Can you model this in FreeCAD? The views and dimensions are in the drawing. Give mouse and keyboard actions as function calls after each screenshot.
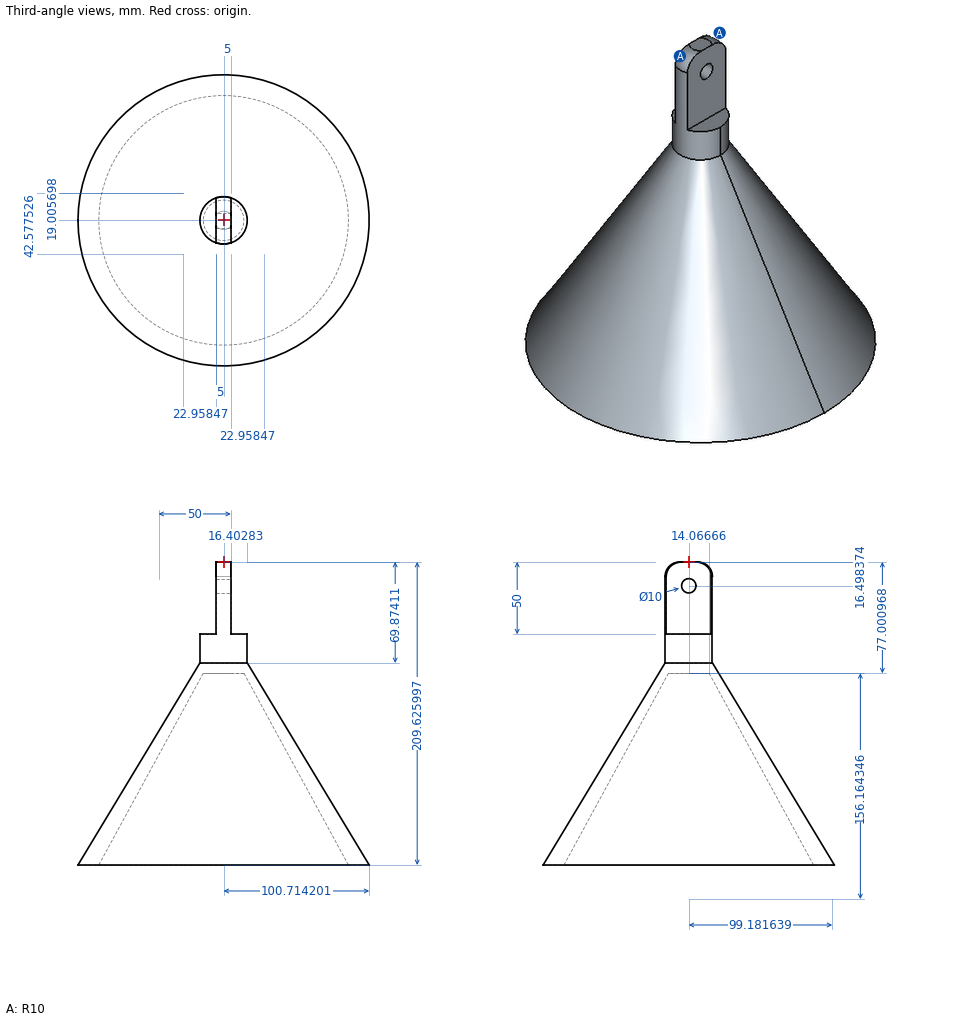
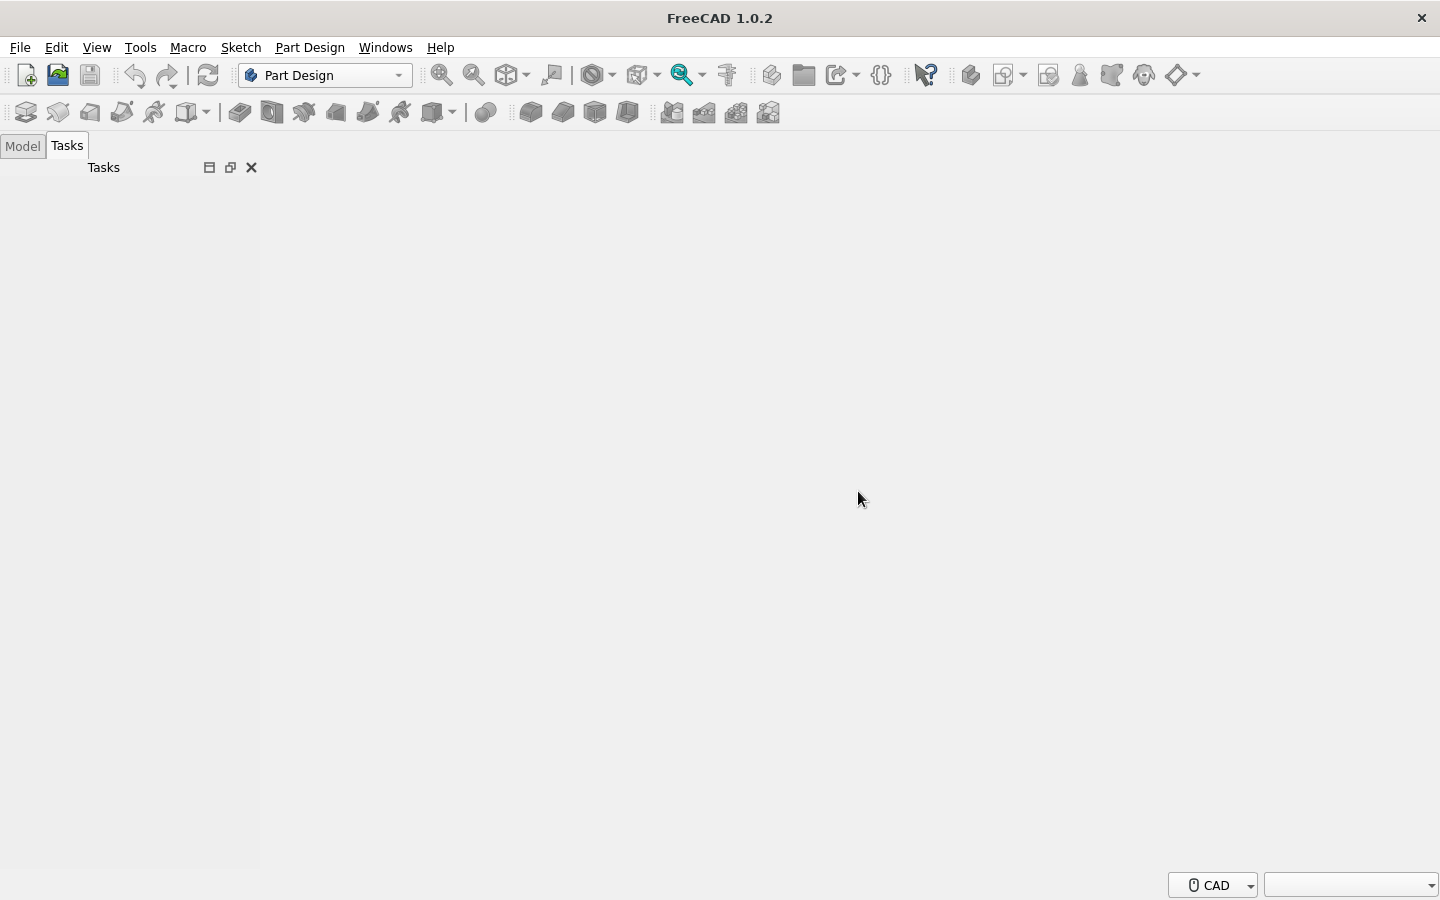
click(26, 76)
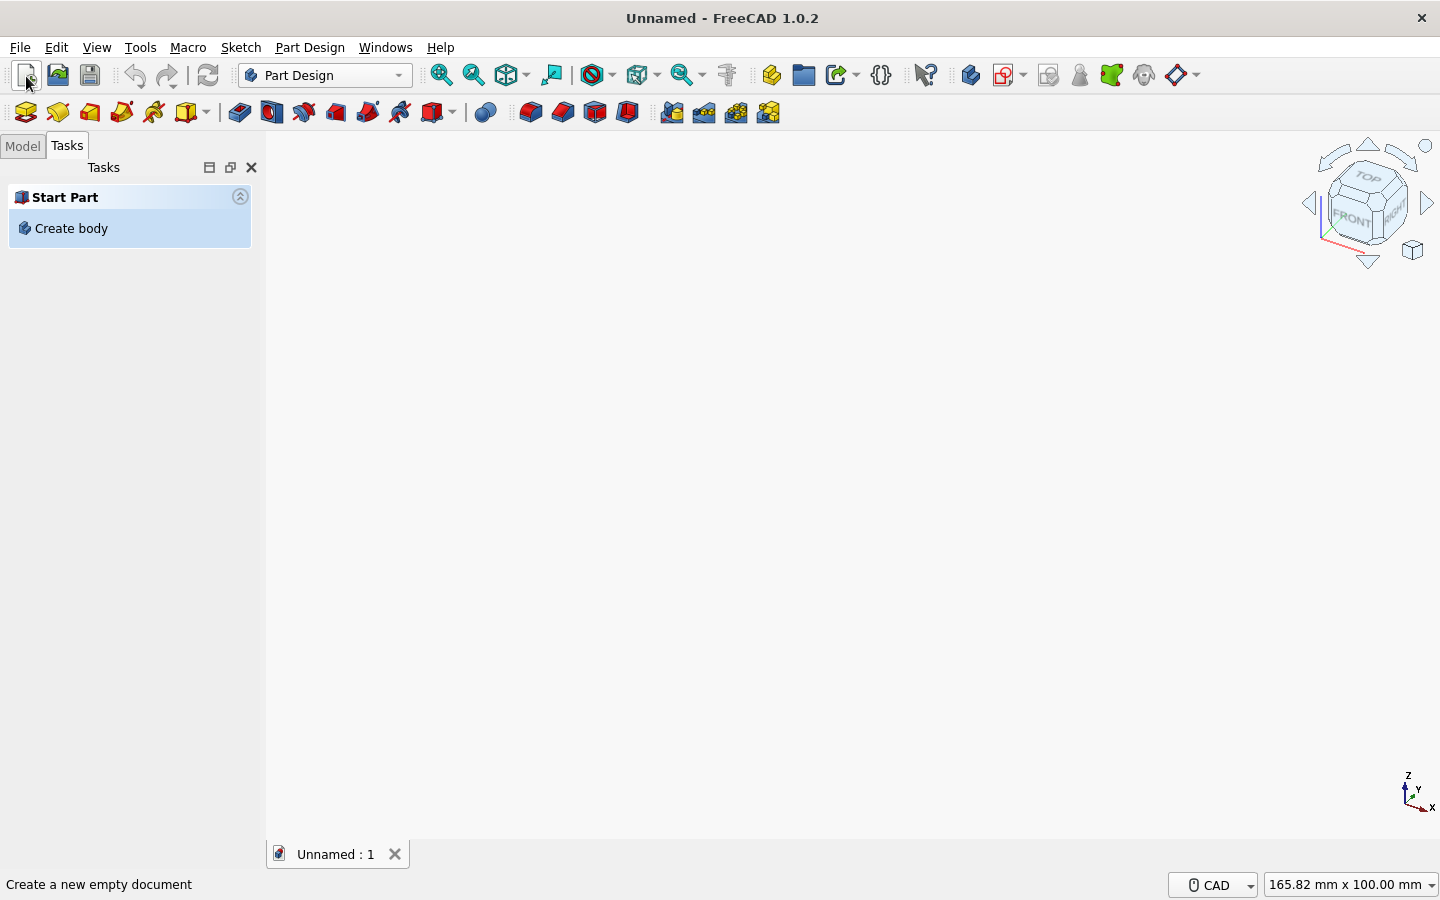
click(1004, 76)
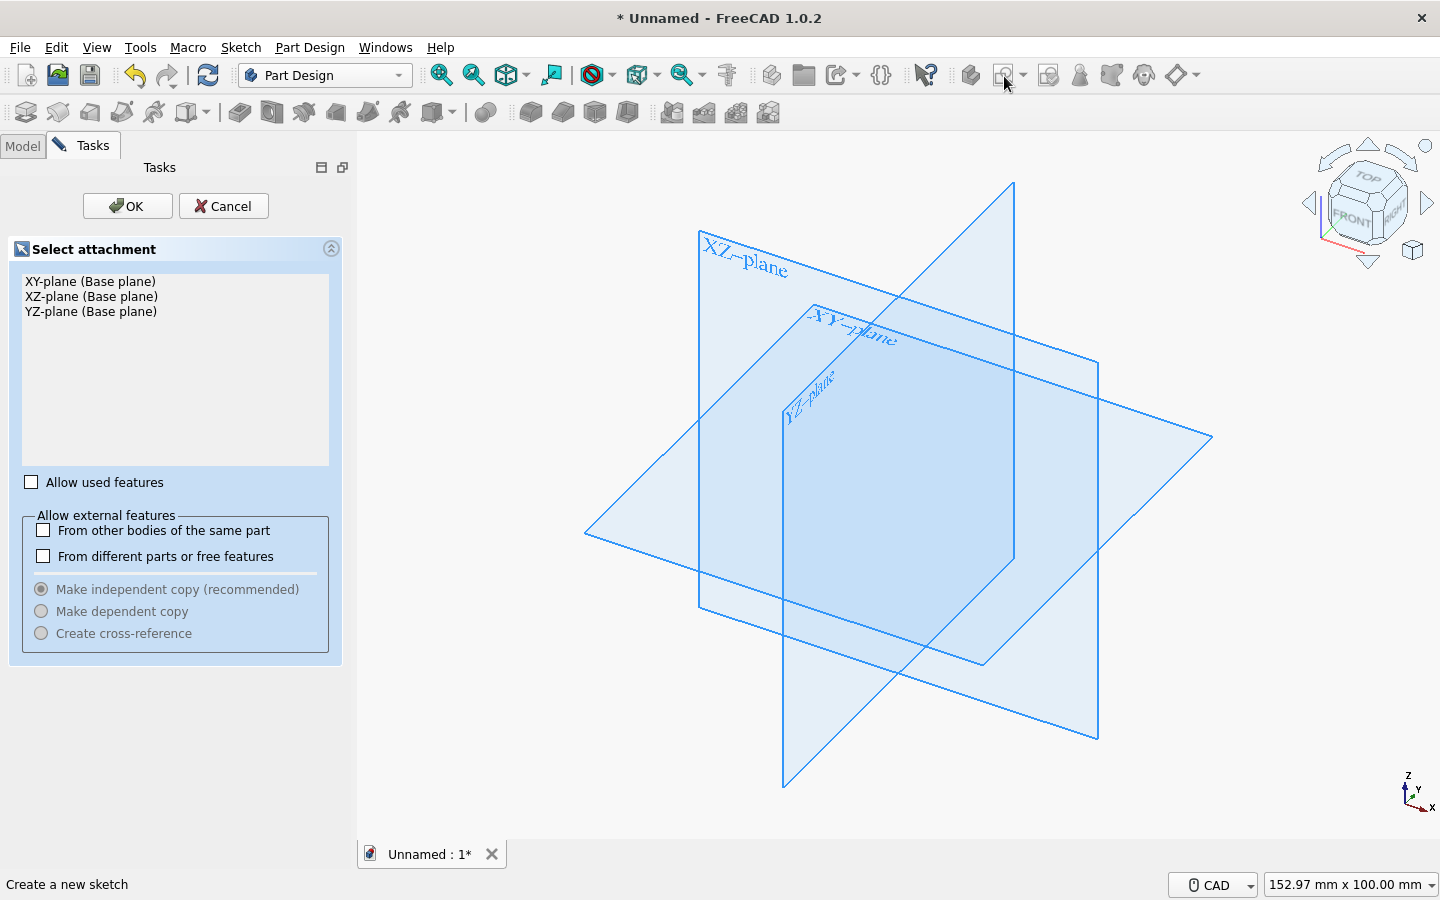
click(82, 296)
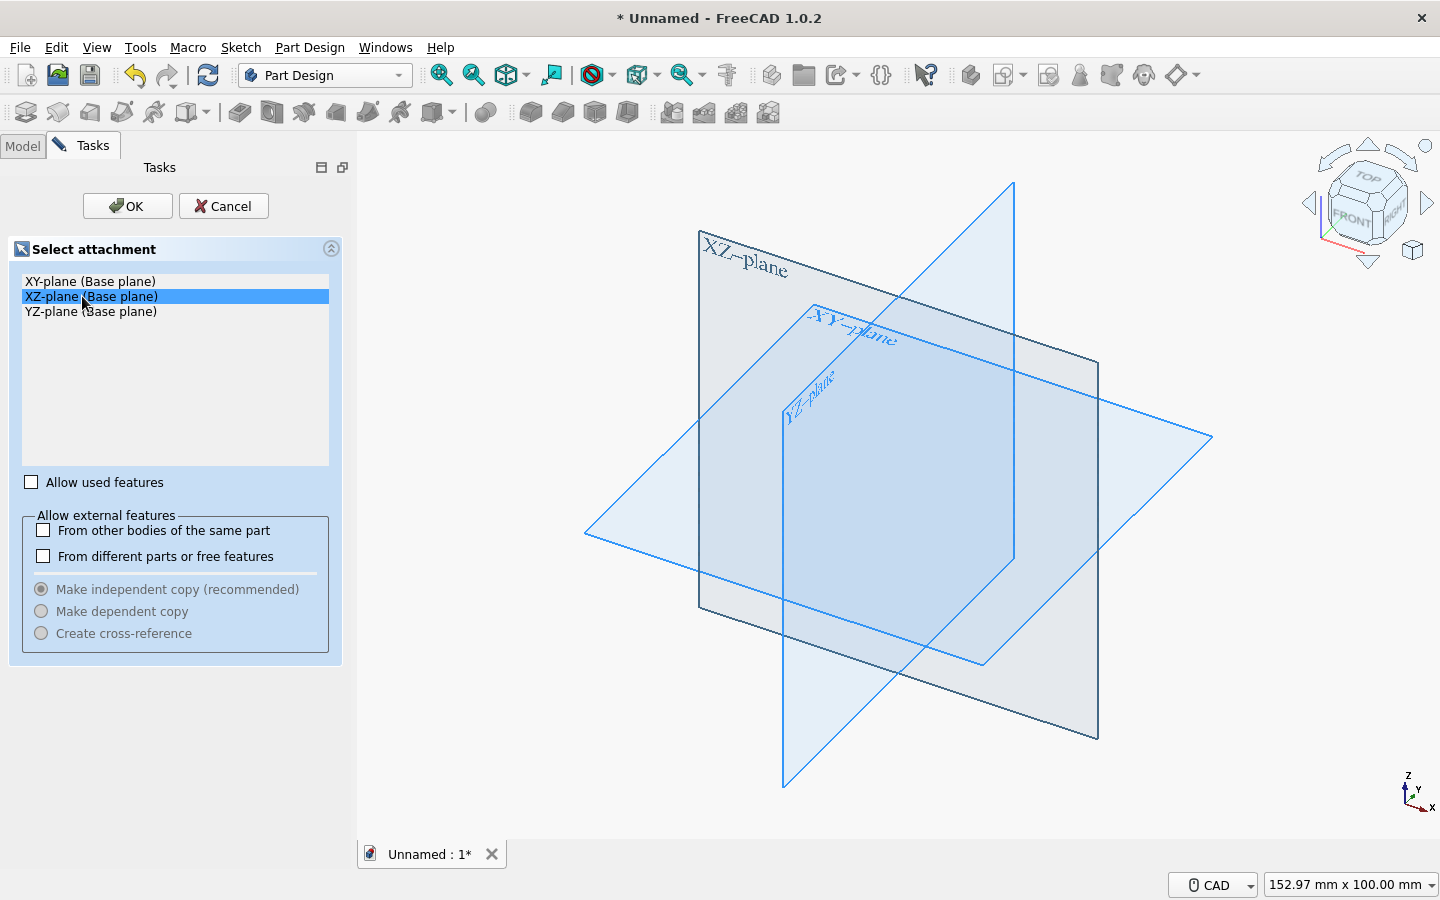
click(128, 206)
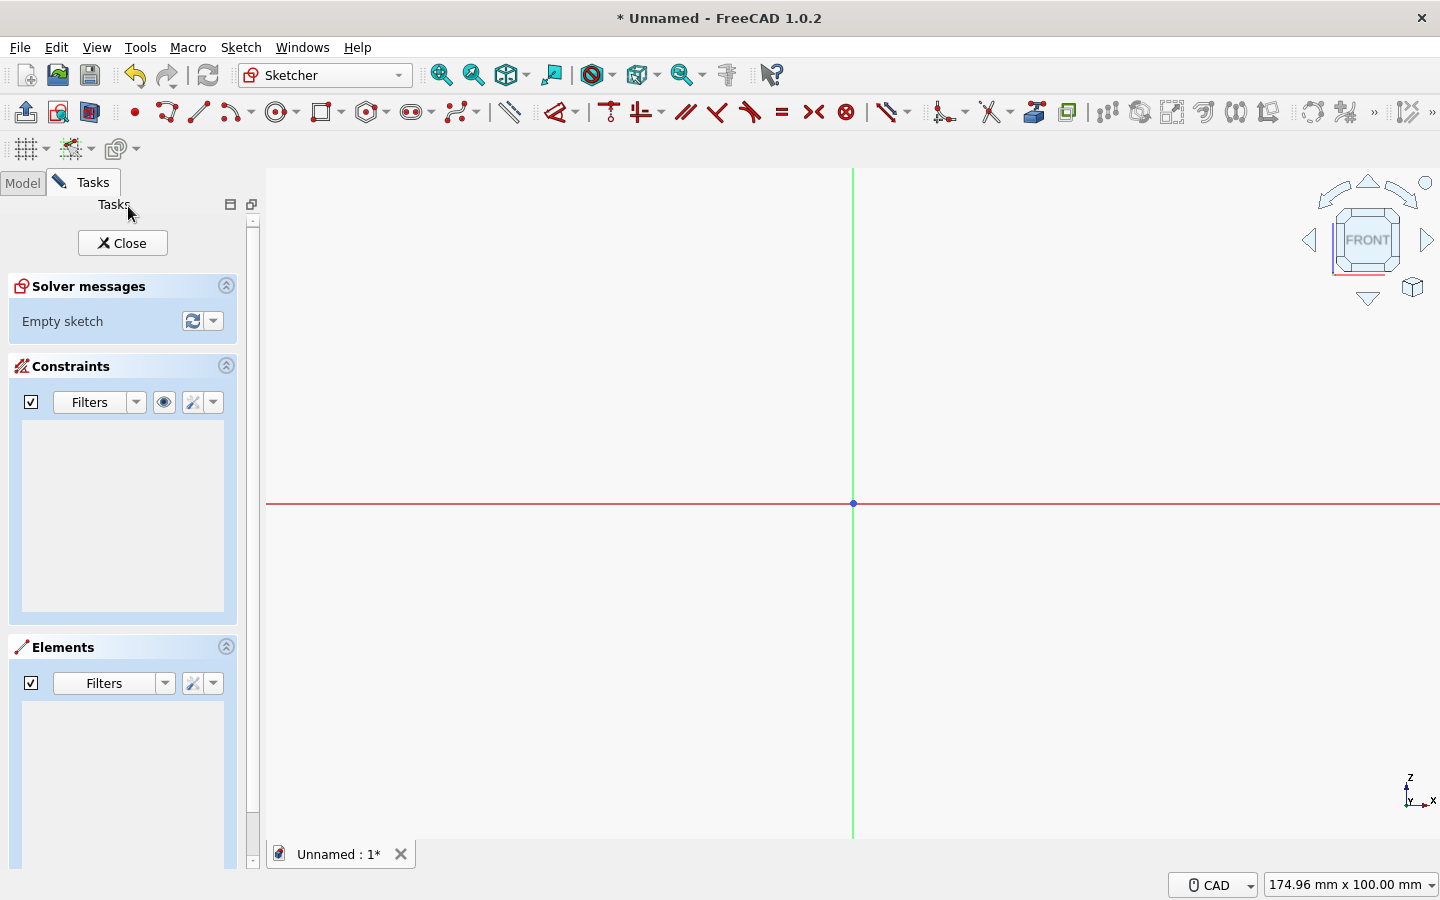
scroll(609, 200, down, 6)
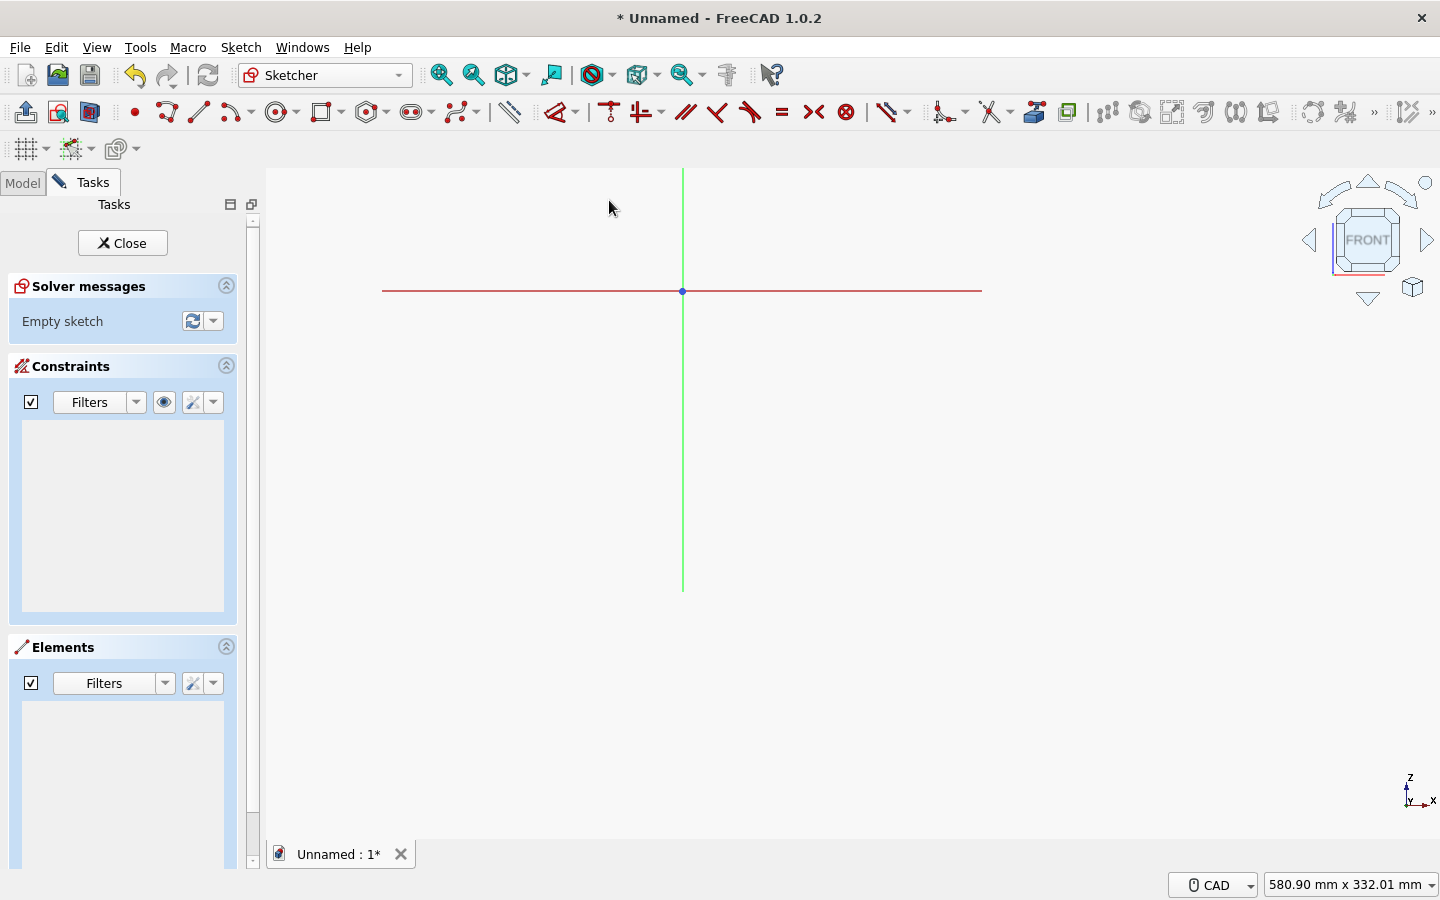
click(168, 112)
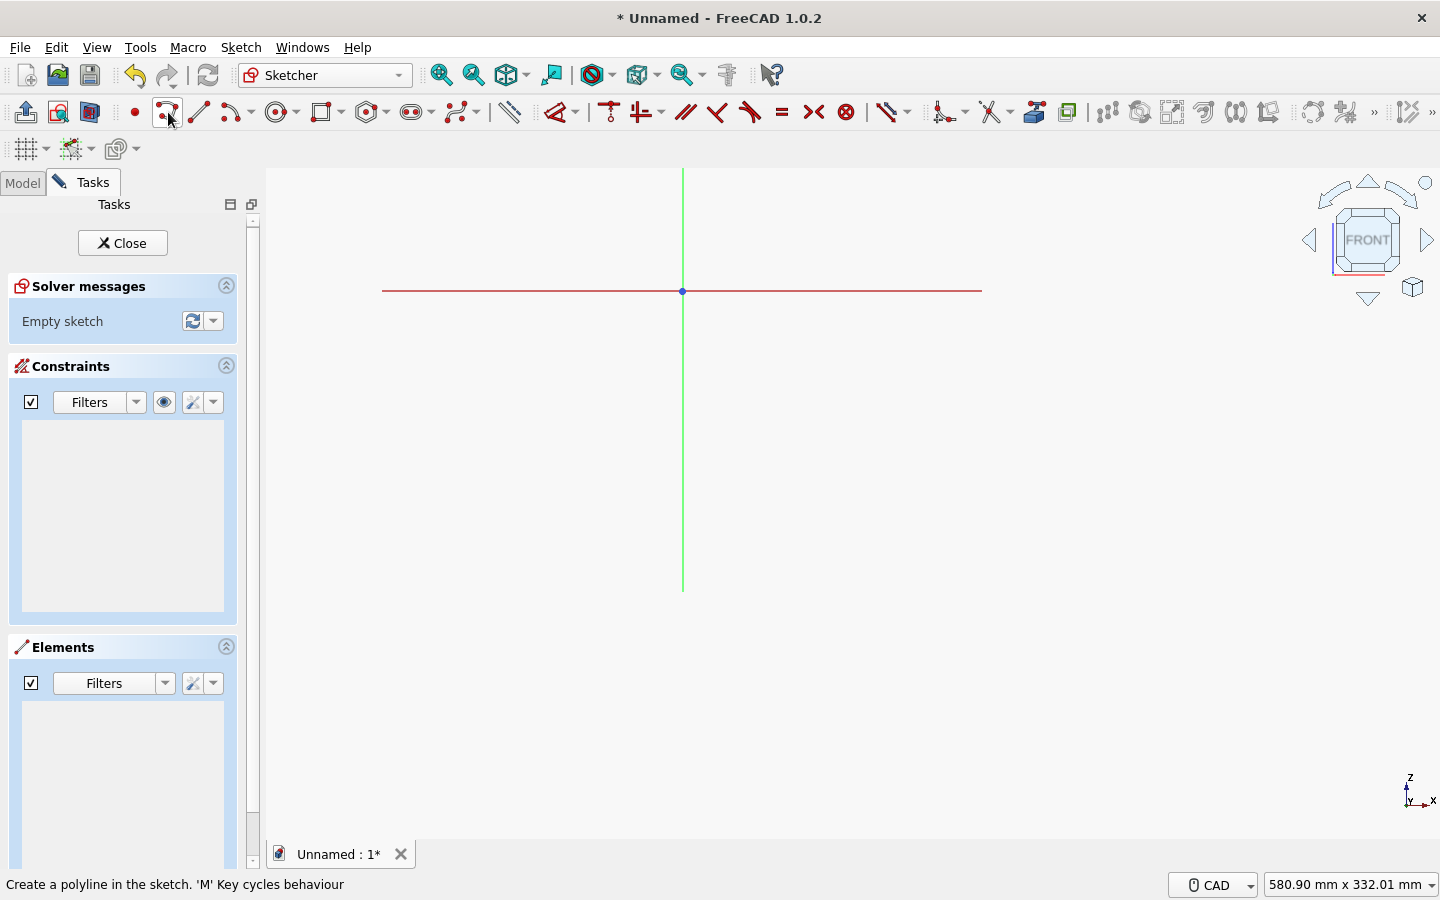
click(683, 291)
click(716, 300)
click(716, 433)
click(886, 715)
click(692, 715)
click(683, 291)
key(Escape)
key(Escape)